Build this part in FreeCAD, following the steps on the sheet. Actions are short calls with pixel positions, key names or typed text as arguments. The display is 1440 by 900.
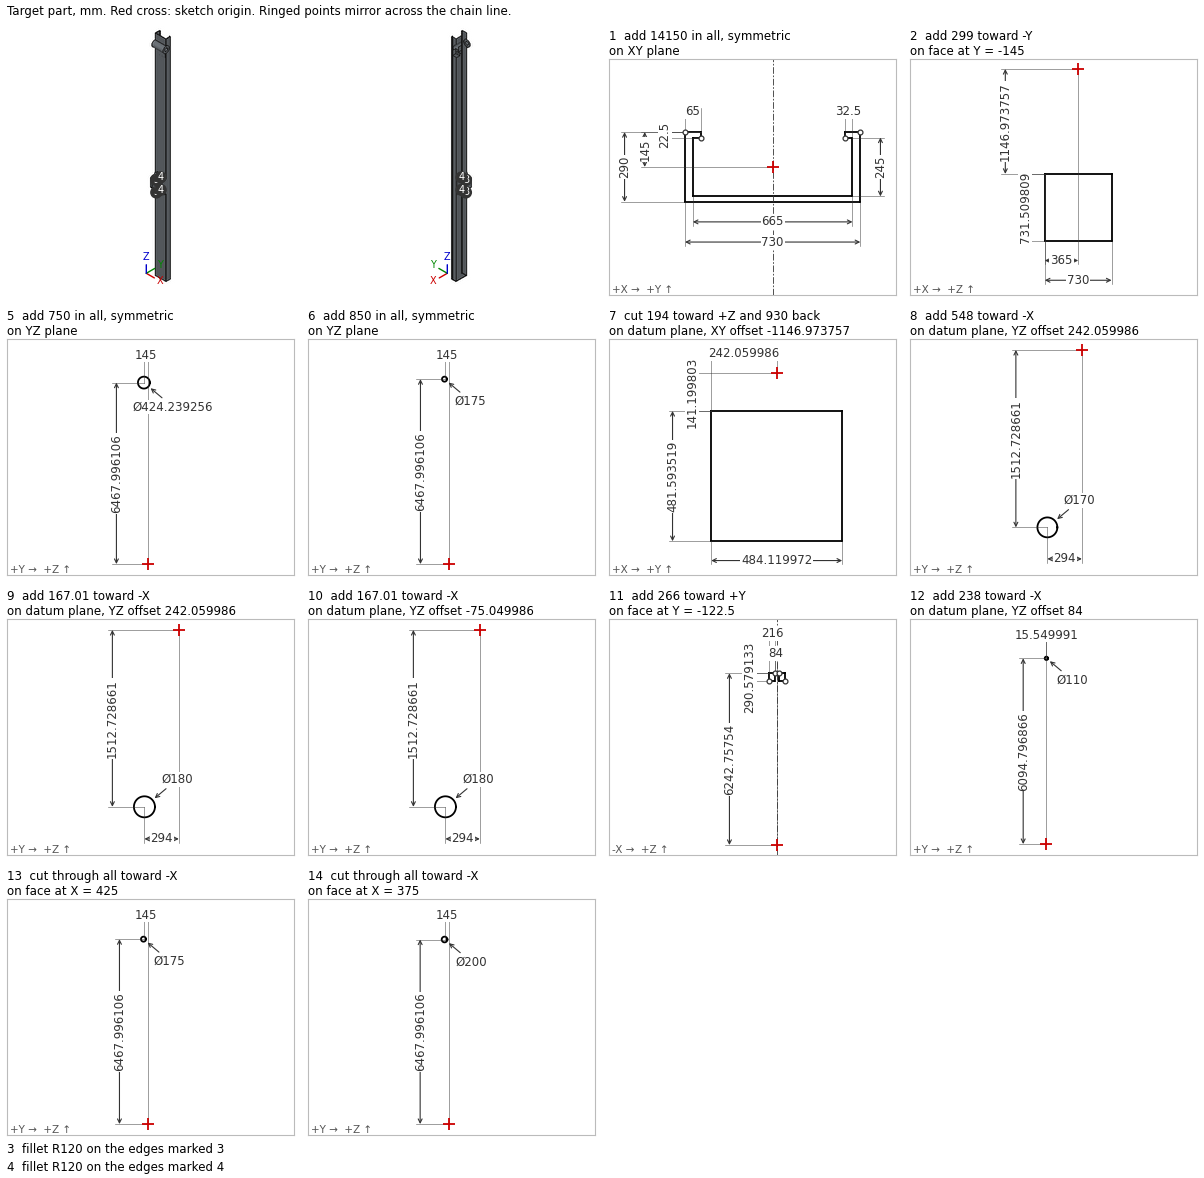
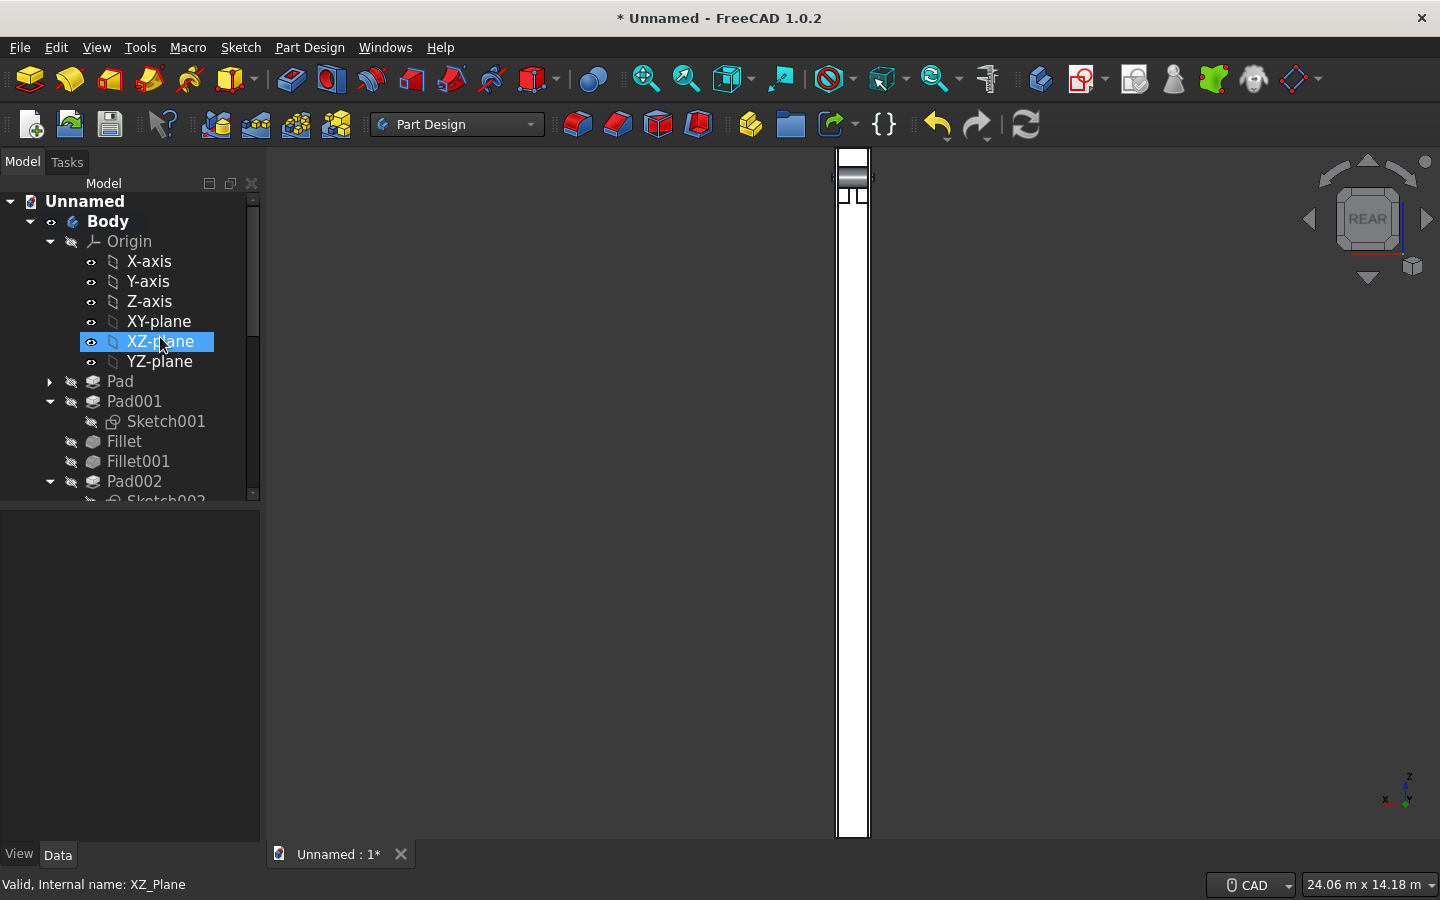
click(136, 362)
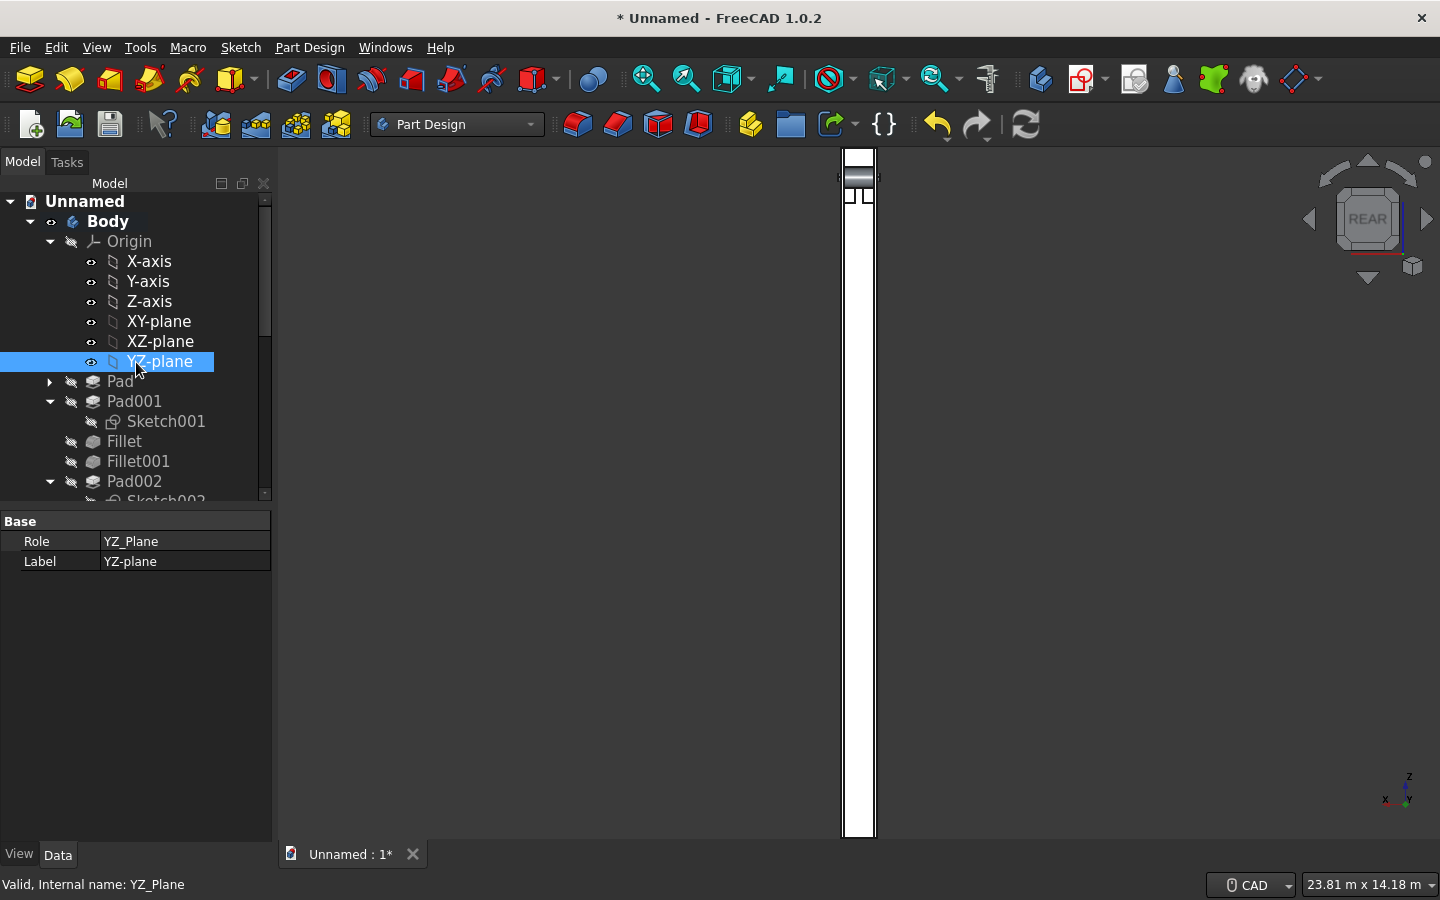
click(1294, 80)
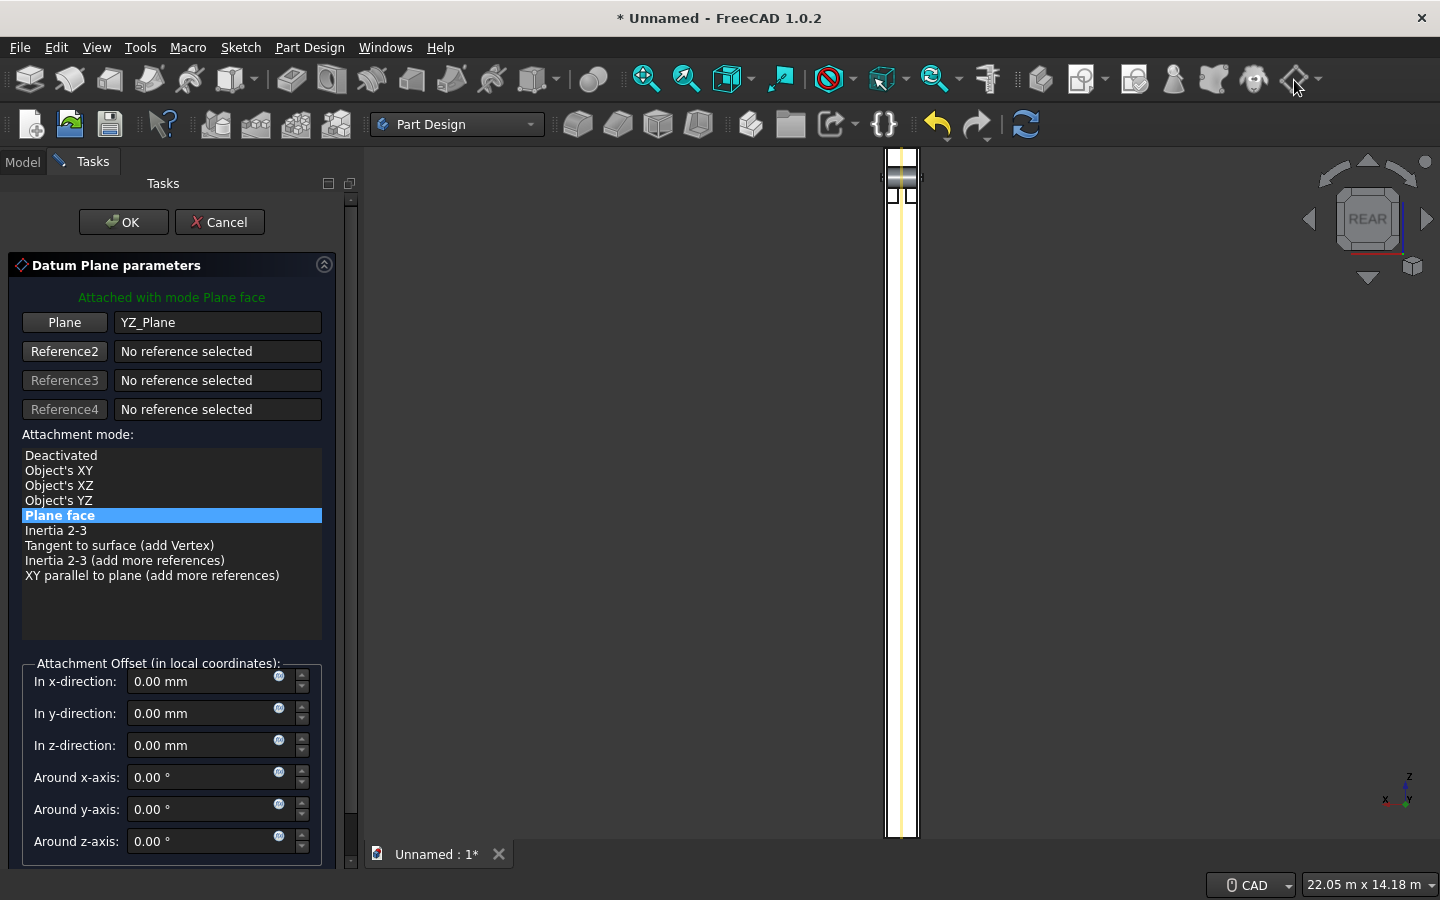
triple_click(210, 745)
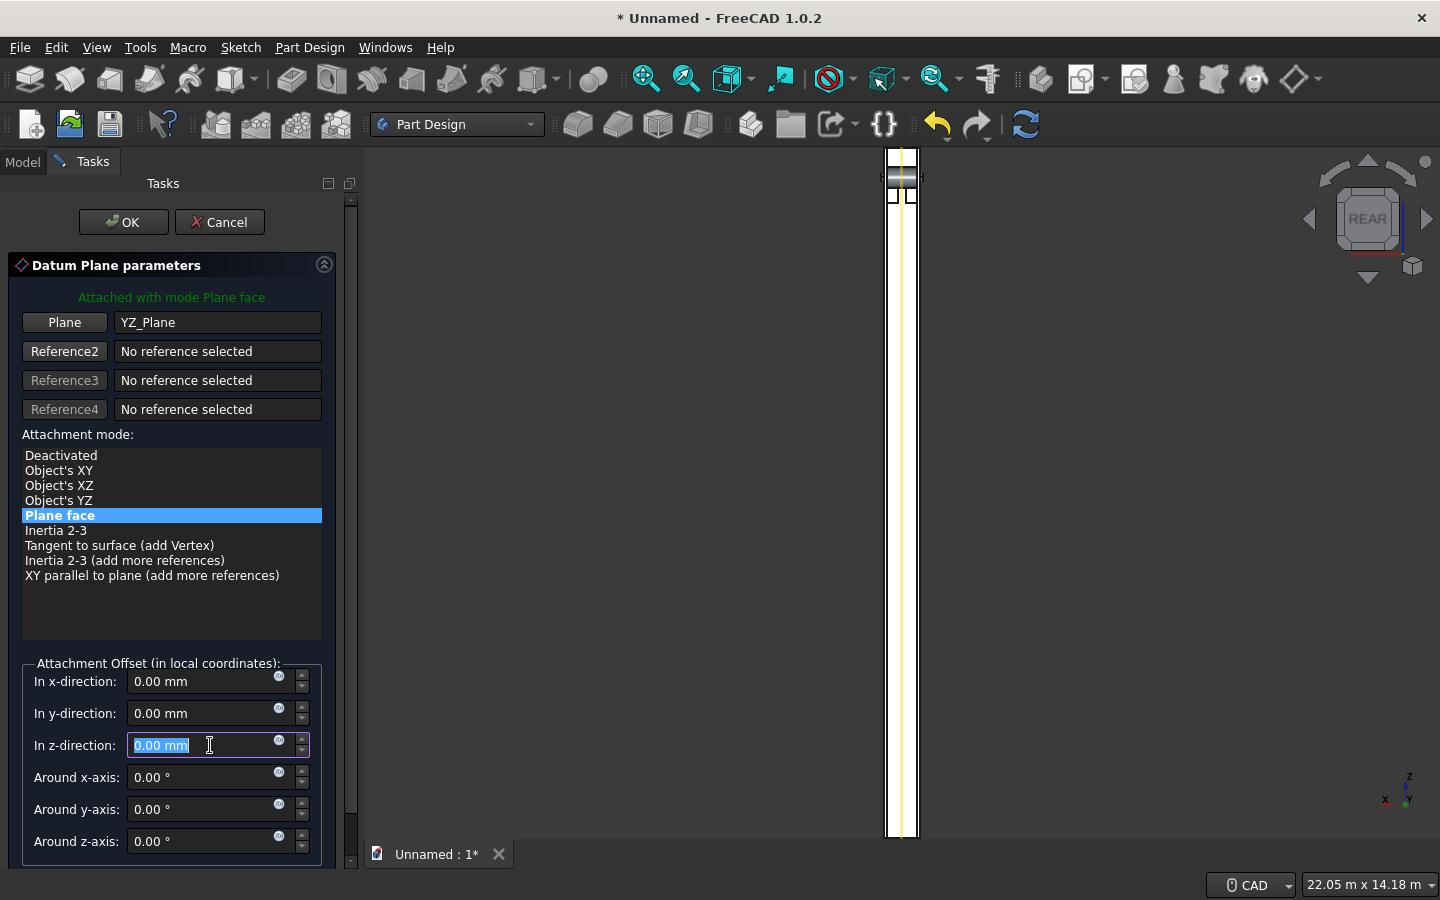
text(84)
key(Tab)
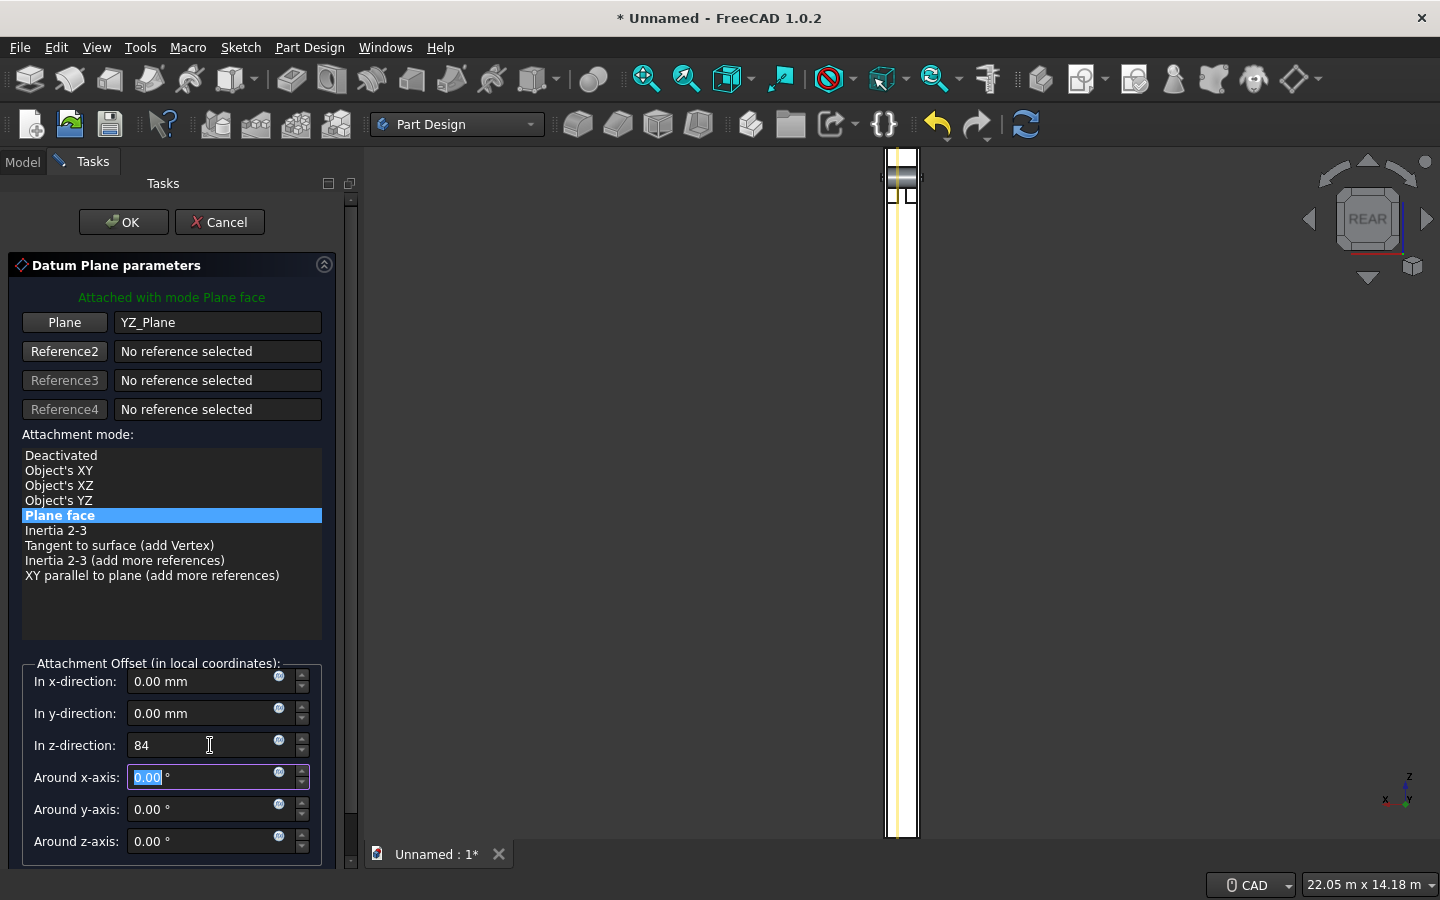
click(124, 222)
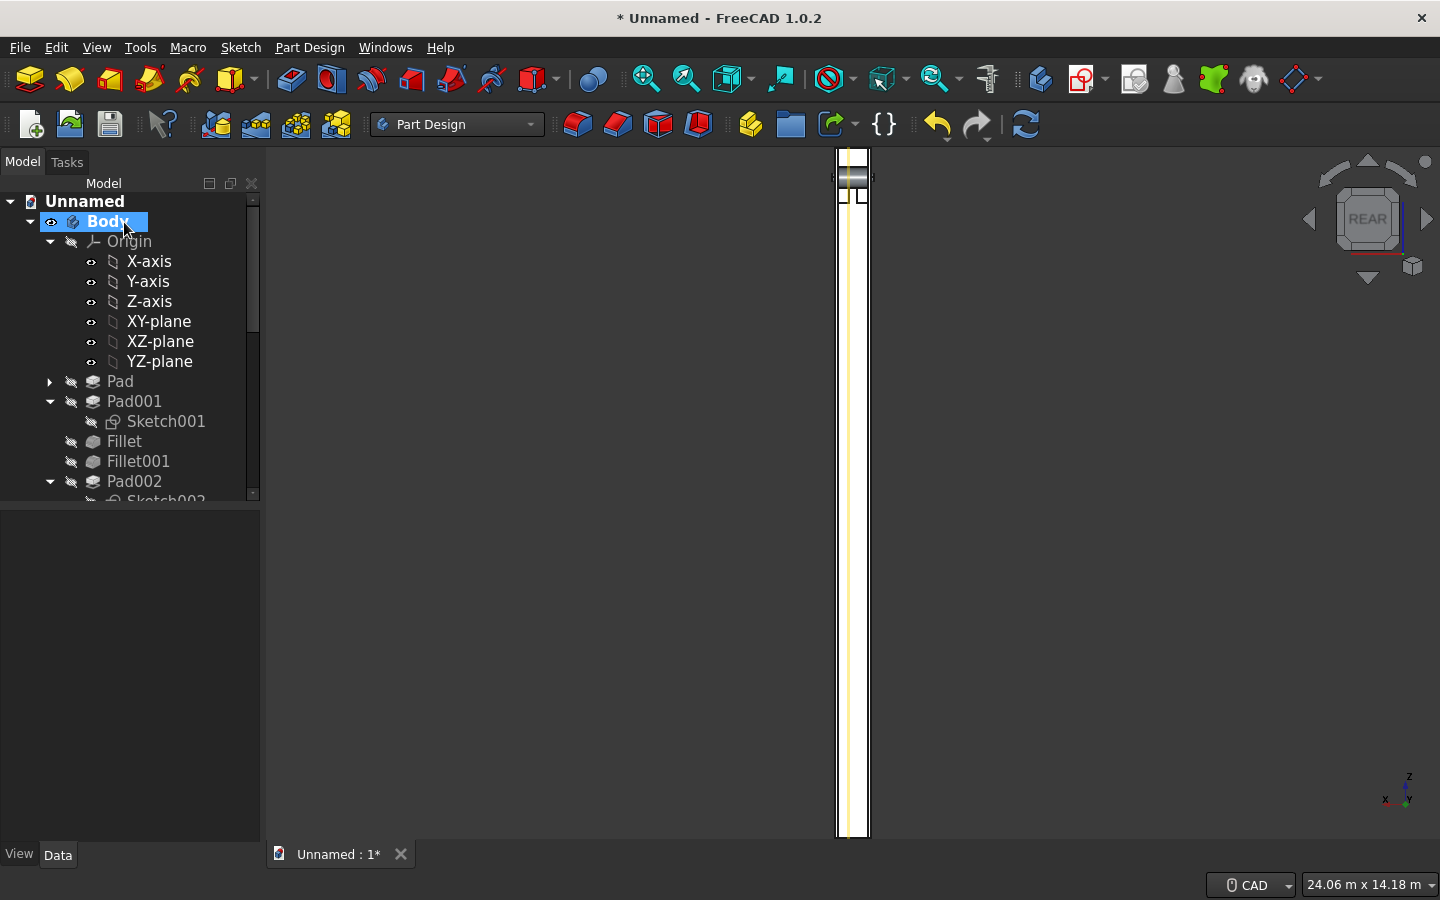
scroll(100, 337, down, 3)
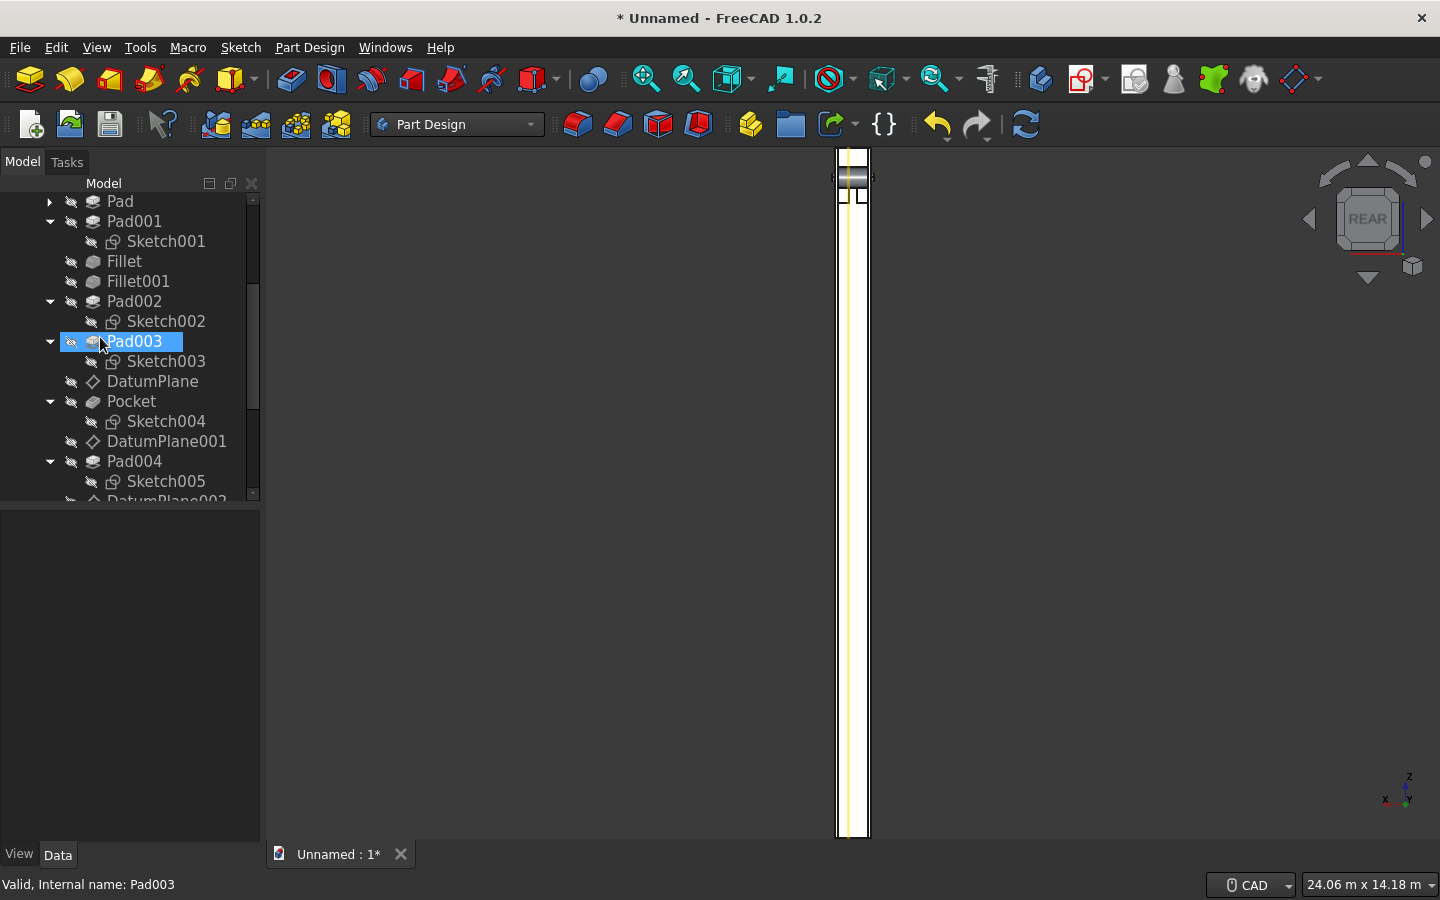
scroll(140, 337, up, 15)